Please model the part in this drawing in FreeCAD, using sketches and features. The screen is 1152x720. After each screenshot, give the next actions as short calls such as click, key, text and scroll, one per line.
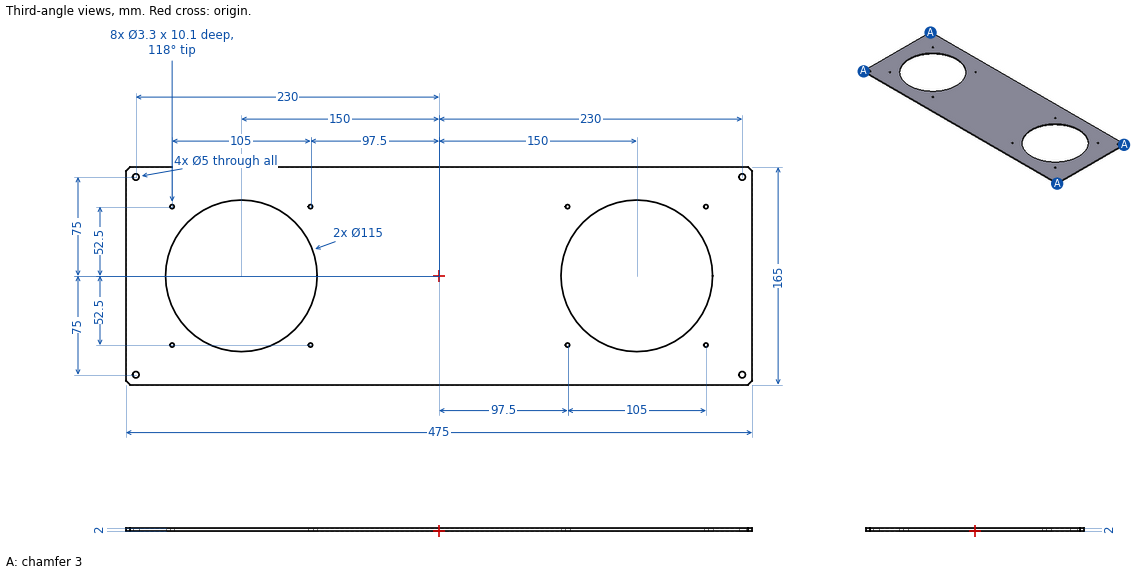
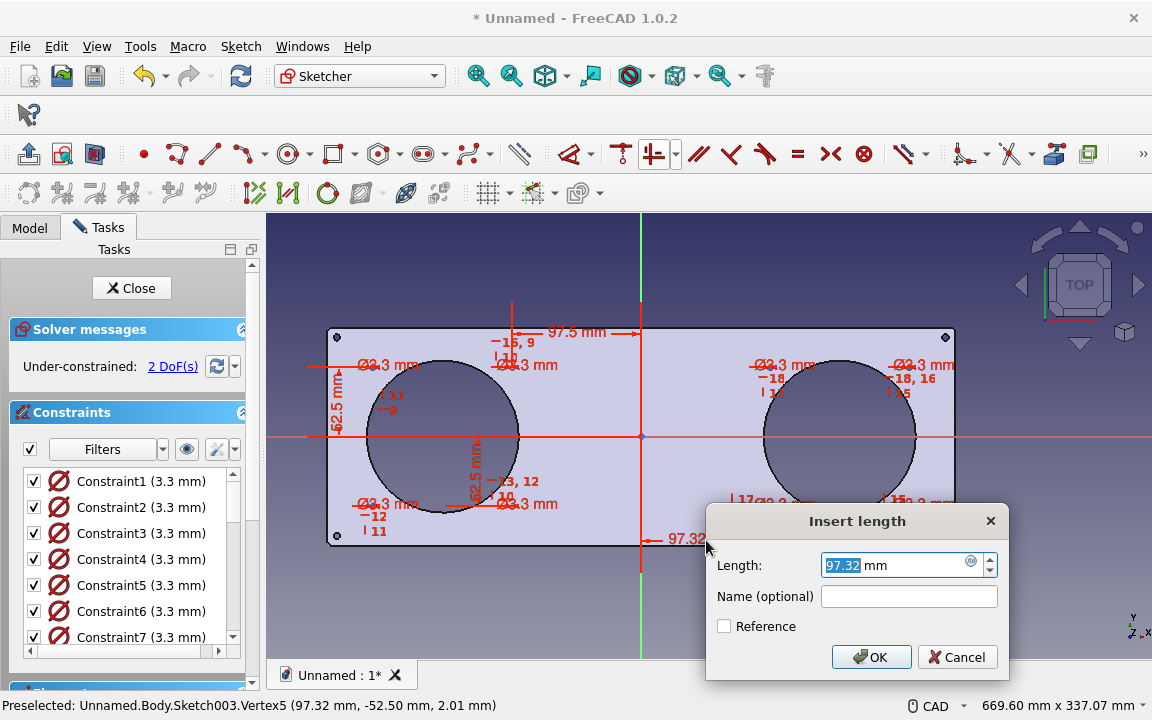
text(97.5)
key(Return)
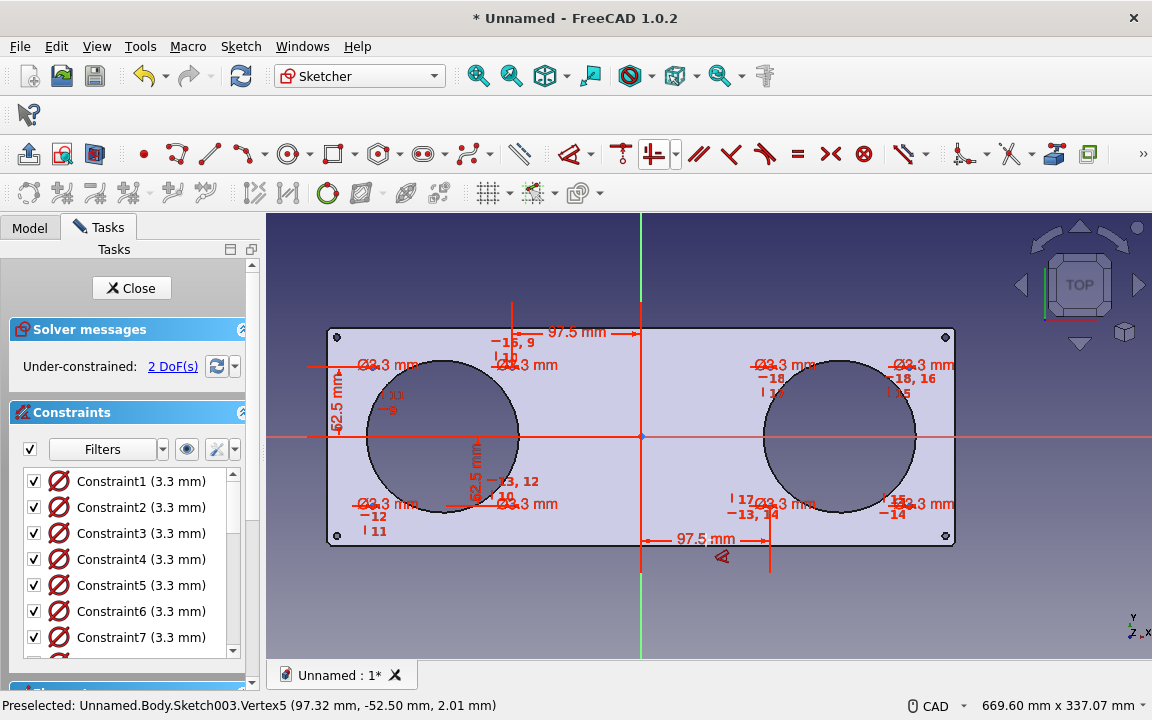
click(373, 367)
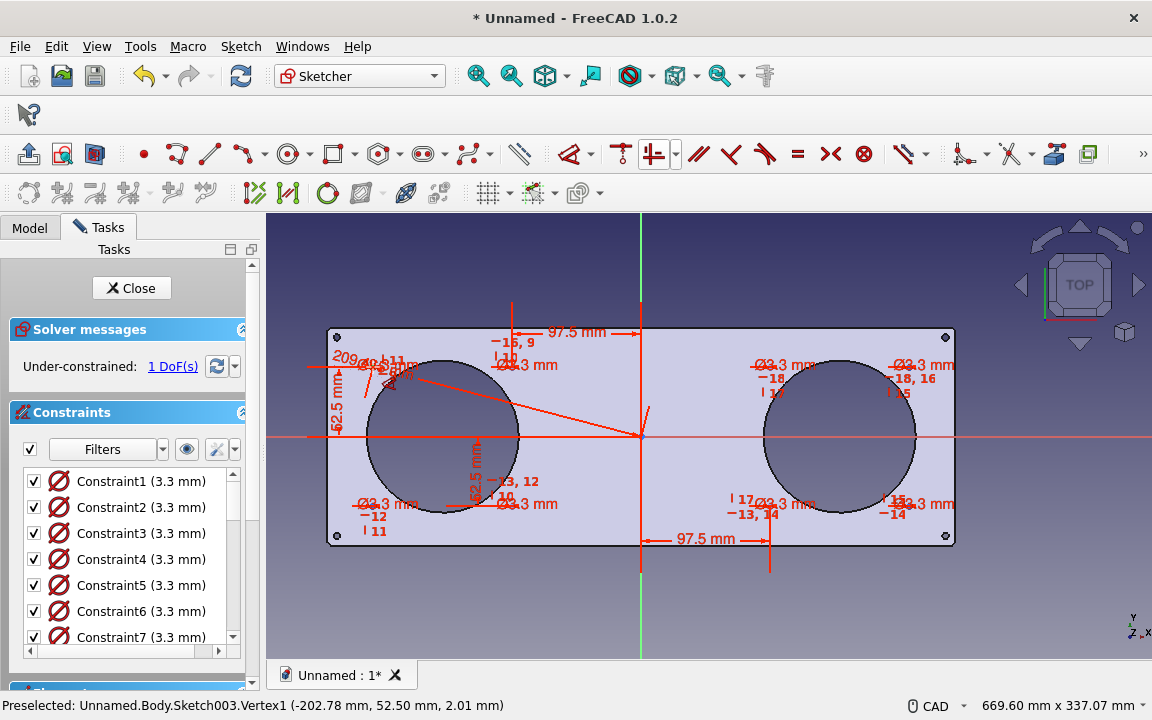
click(512, 367)
click(443, 333)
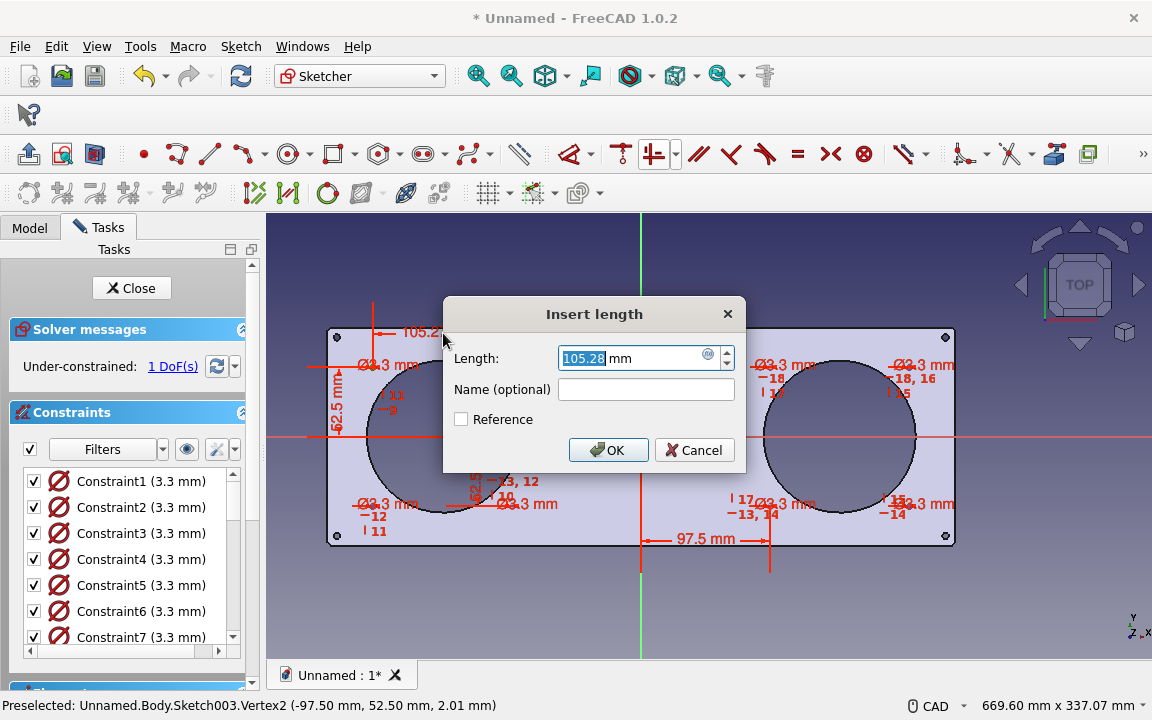
text(105)
key(Return)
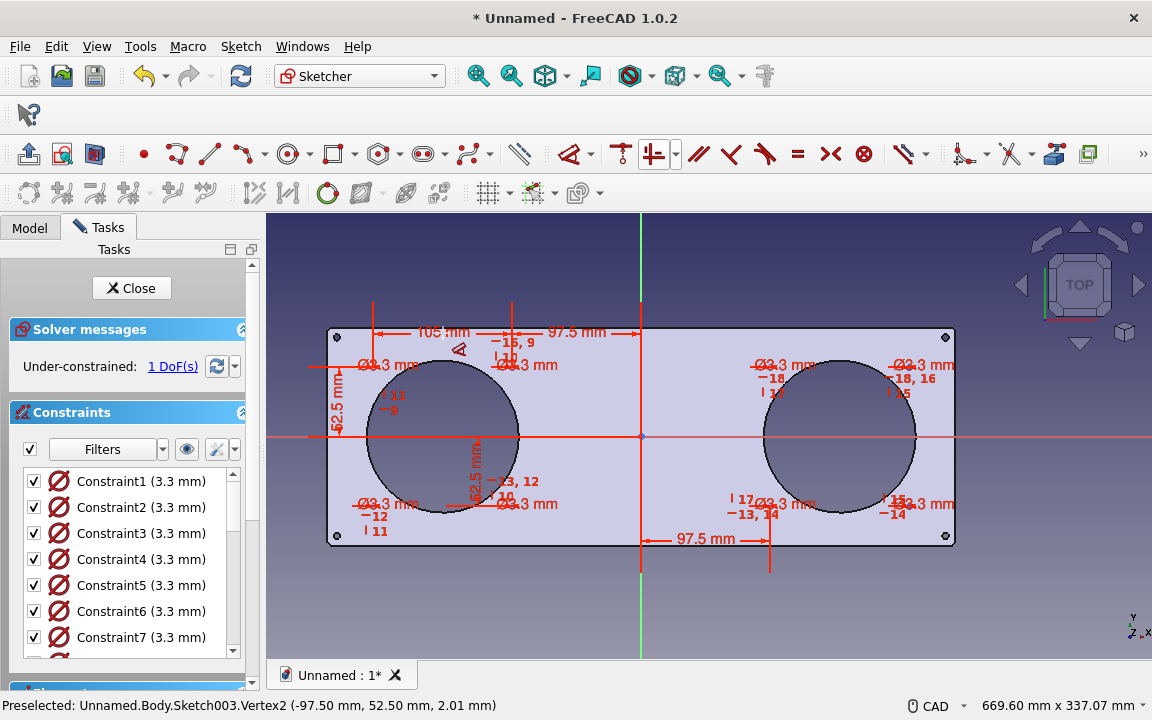
click(770, 506)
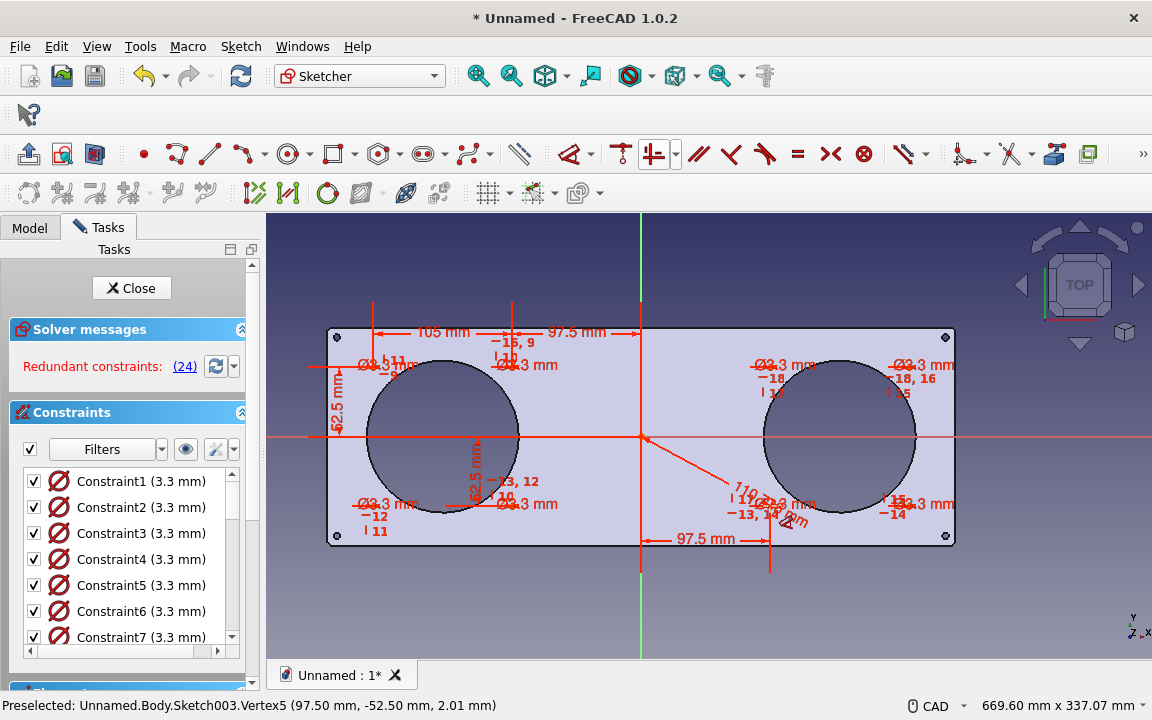
click(909, 506)
click(840, 540)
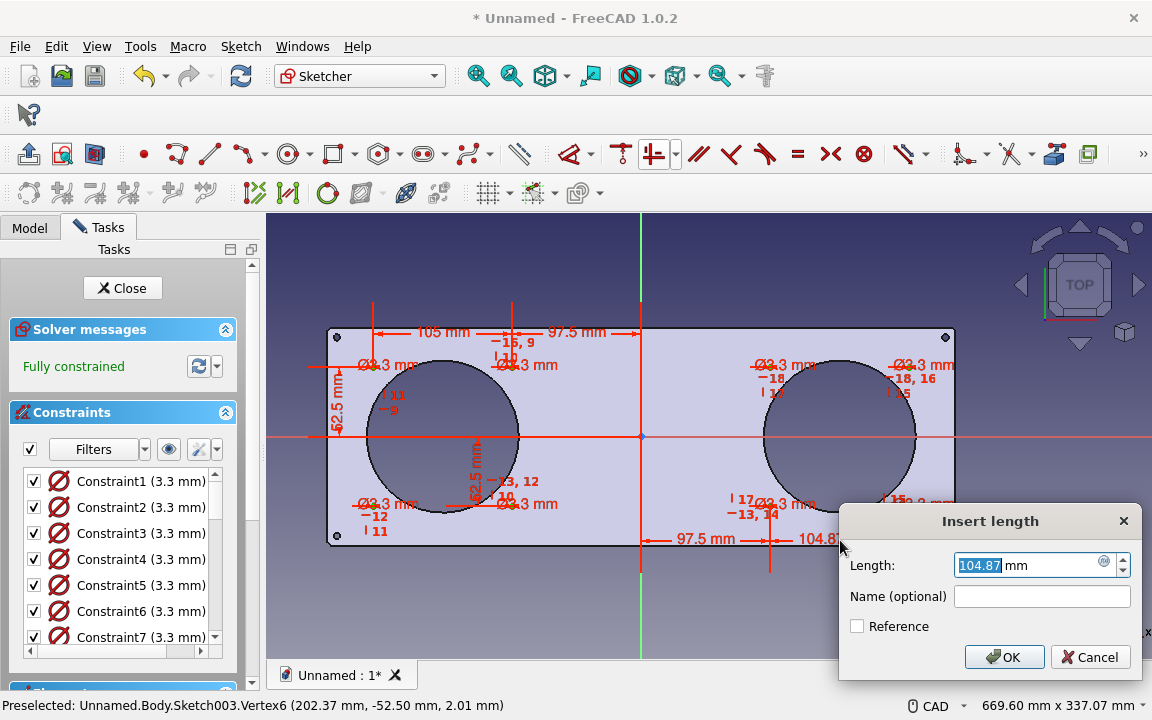
text(105)
key(Return)
key(Escape)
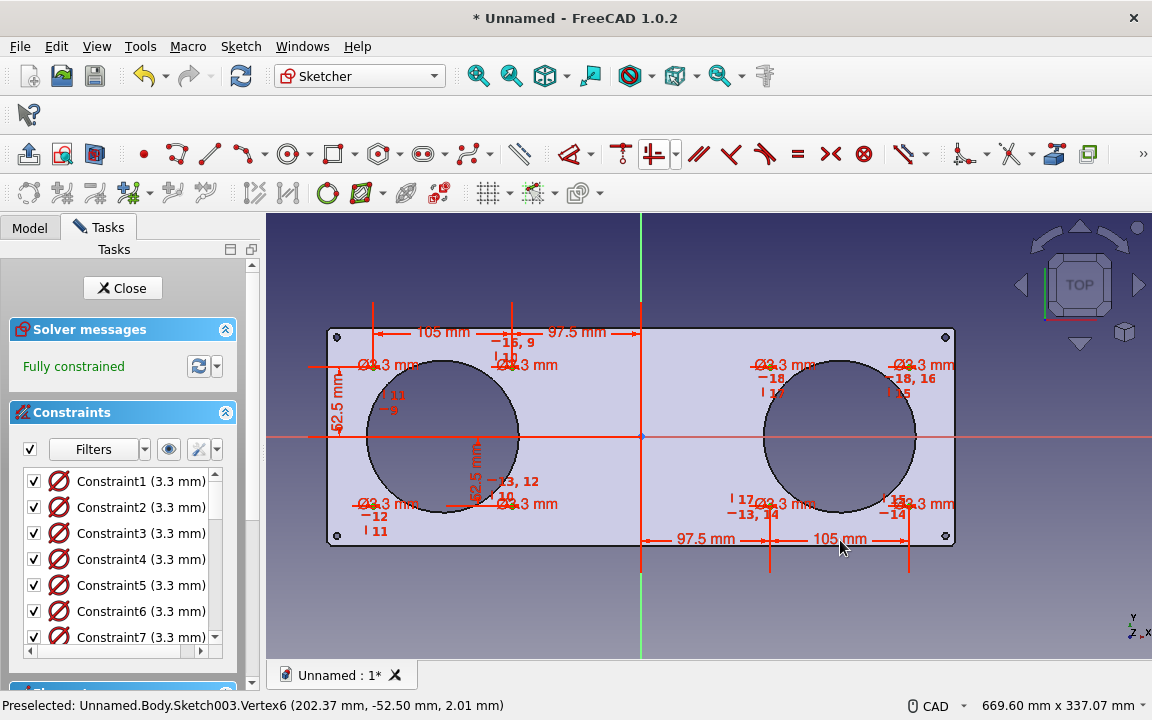
click(123, 288)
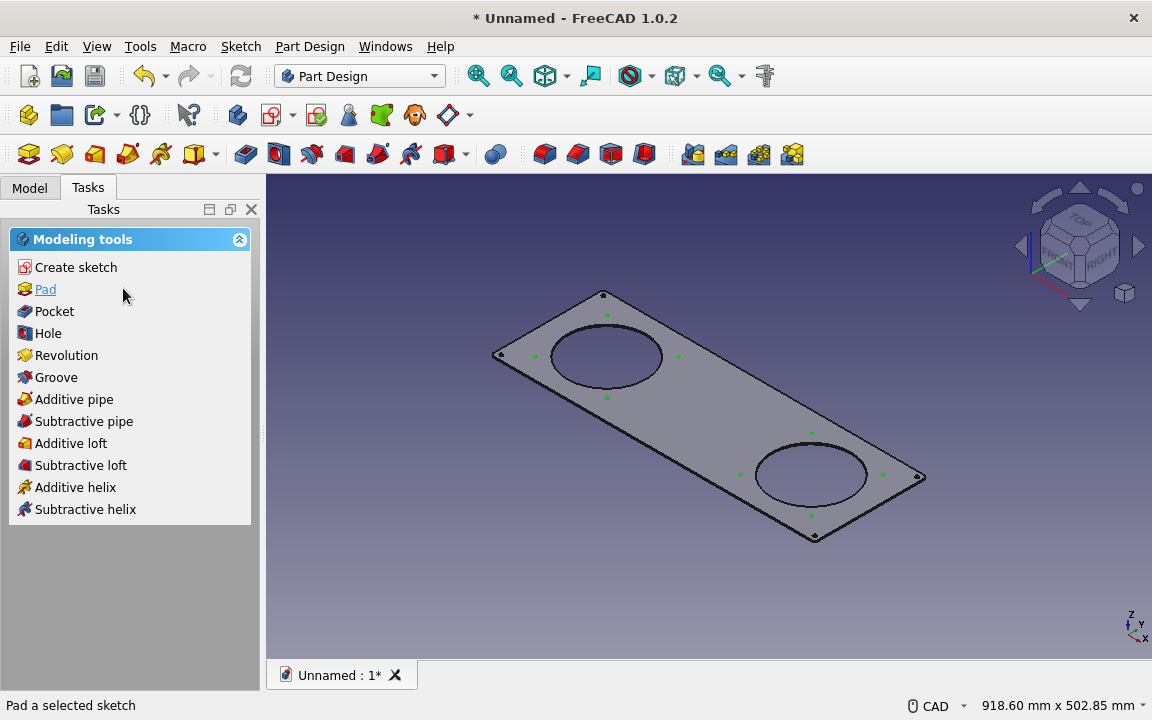
click(279, 154)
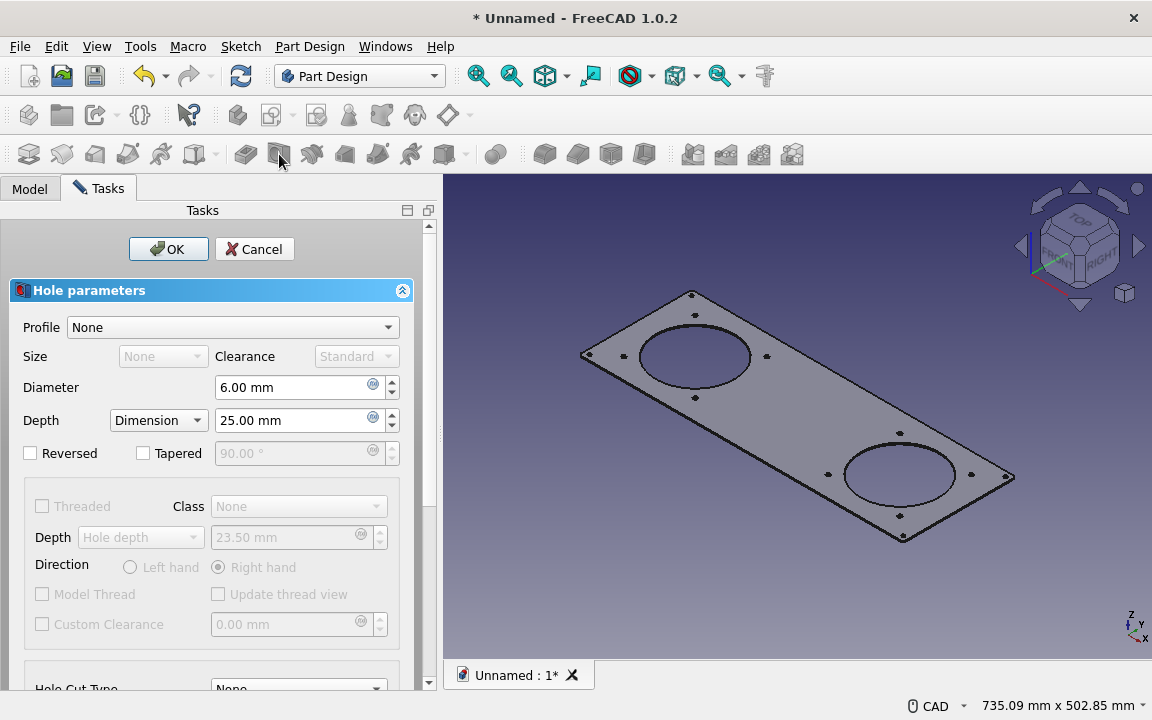
triple_click(300, 388)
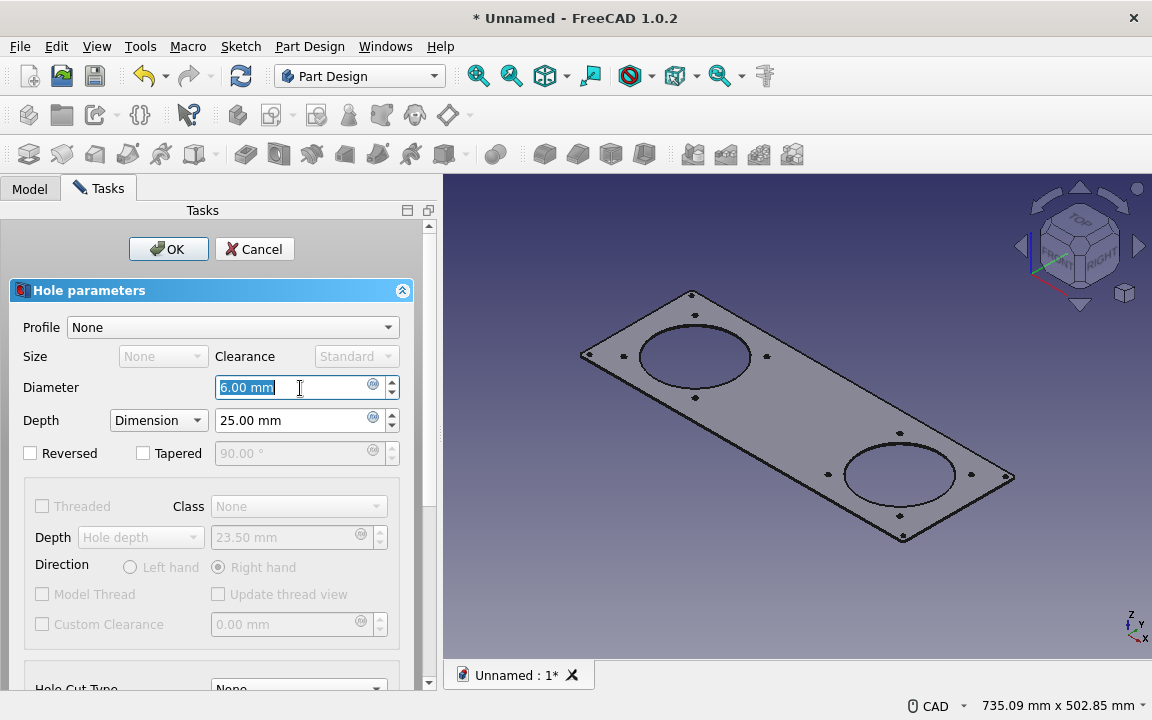
text(3.3)
key(Tab)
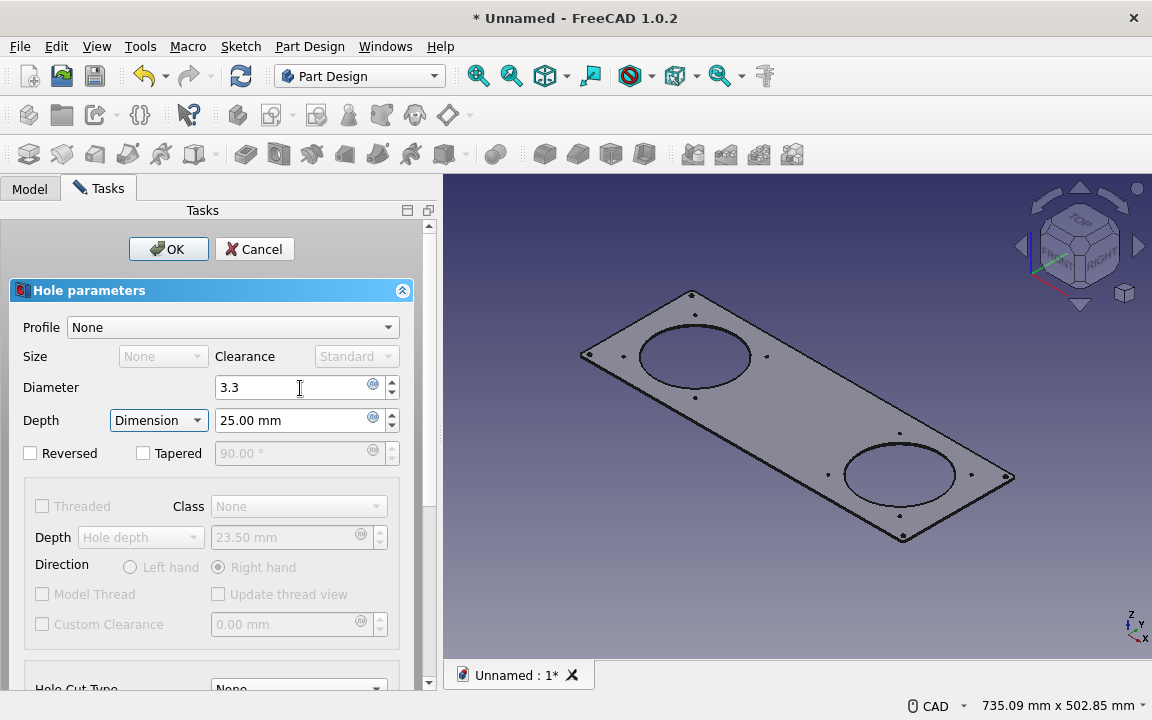
triple_click(300, 420)